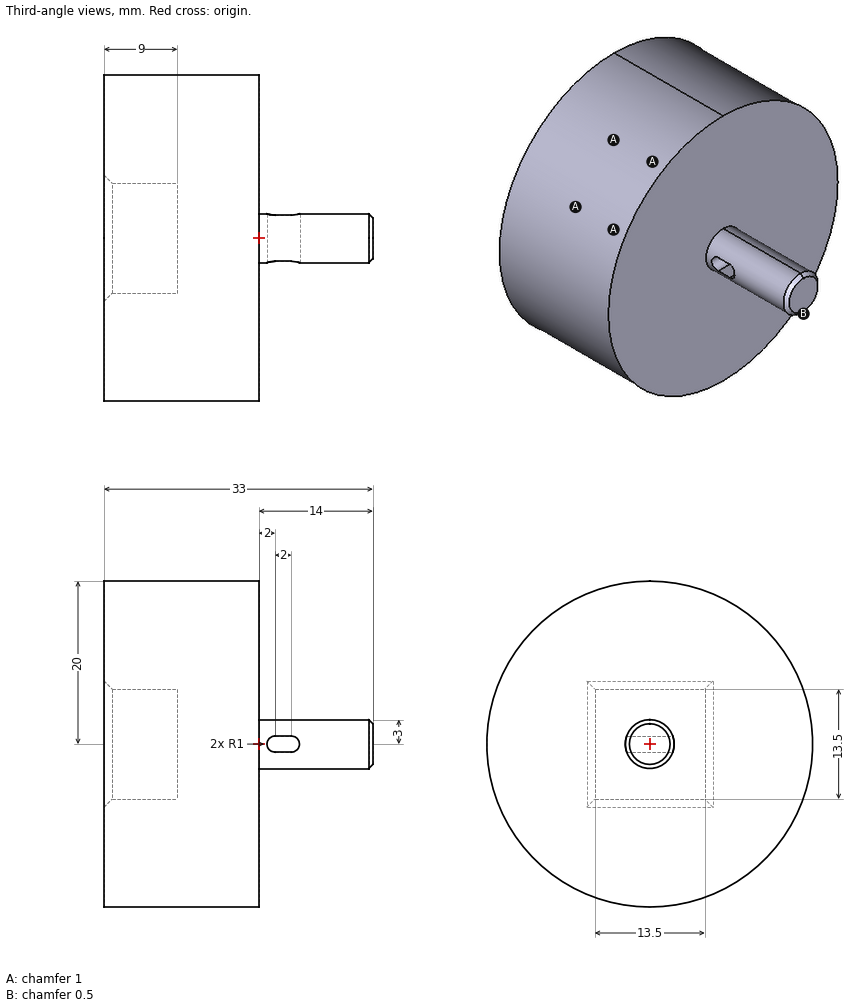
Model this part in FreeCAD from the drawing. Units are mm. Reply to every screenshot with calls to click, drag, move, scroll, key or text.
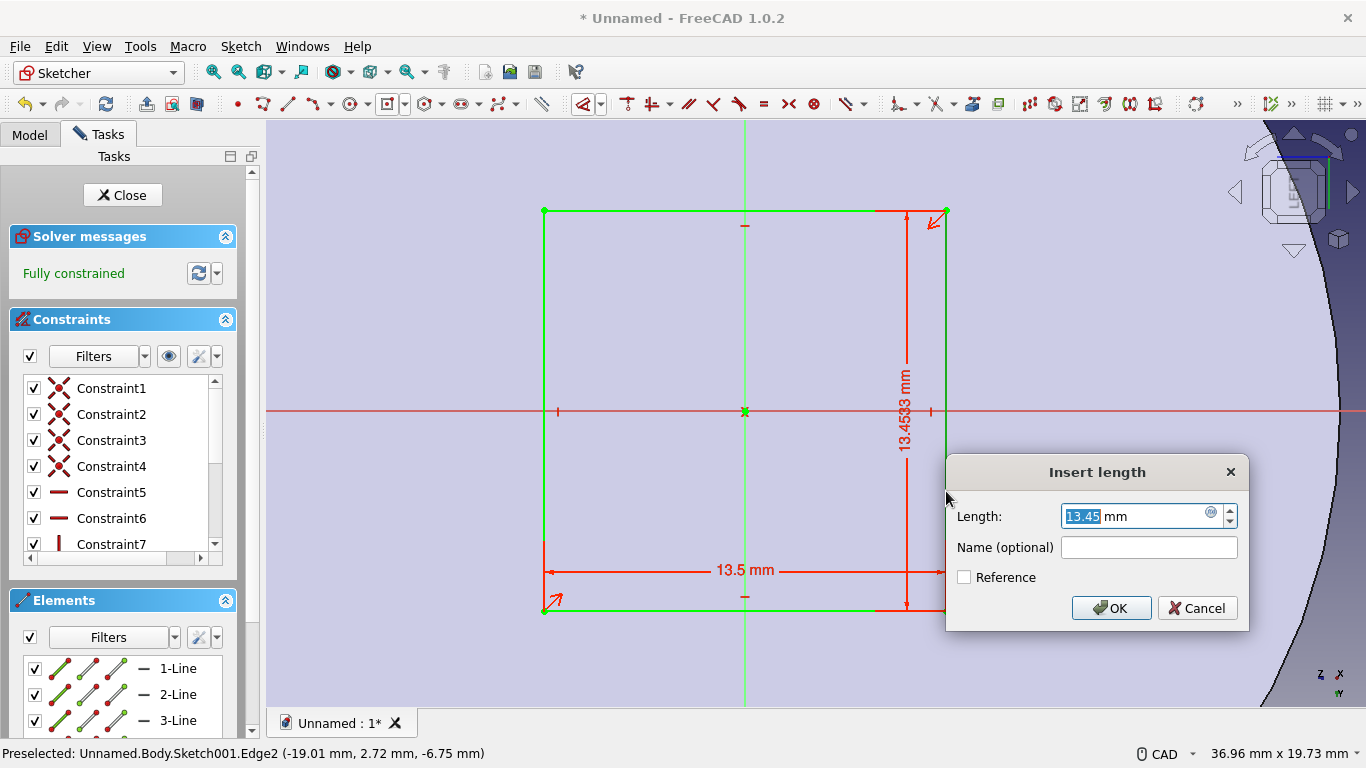
text(13.5)
key(Return)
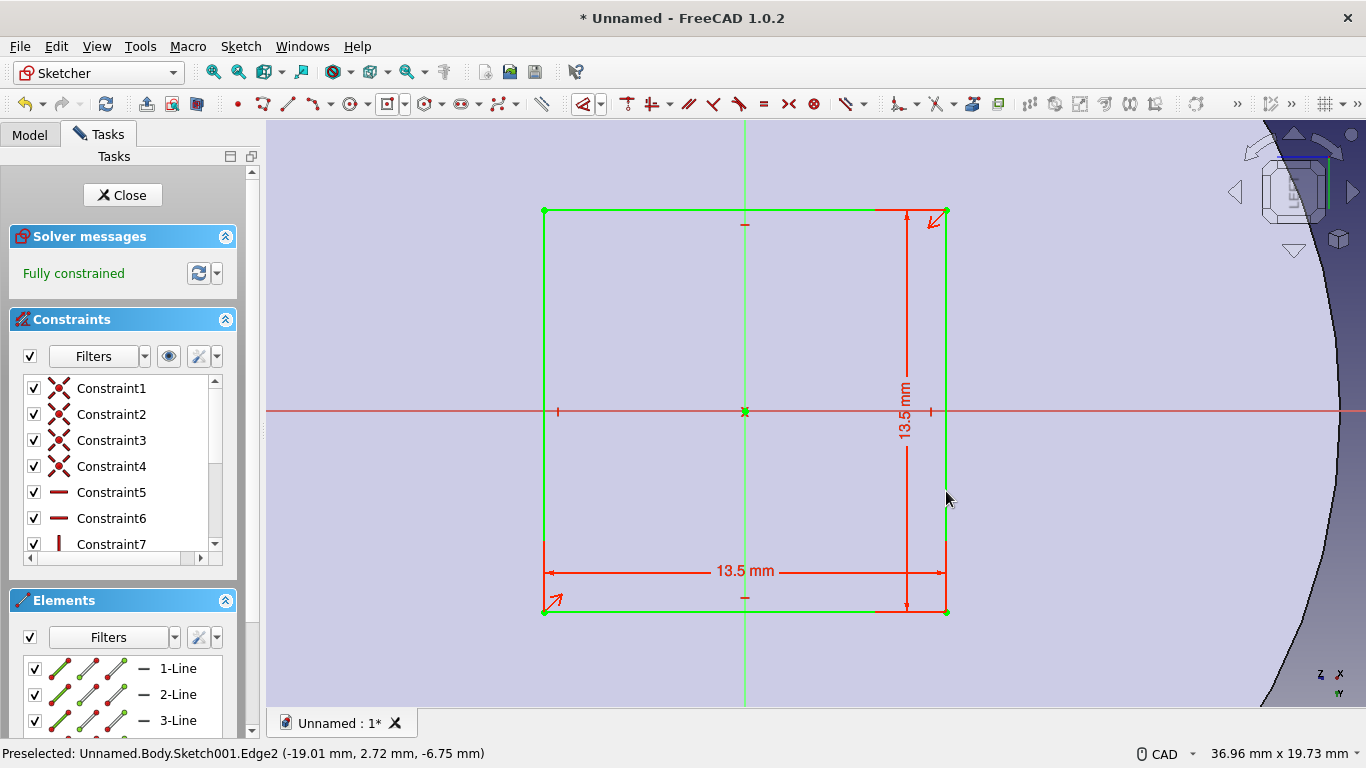
click(123, 195)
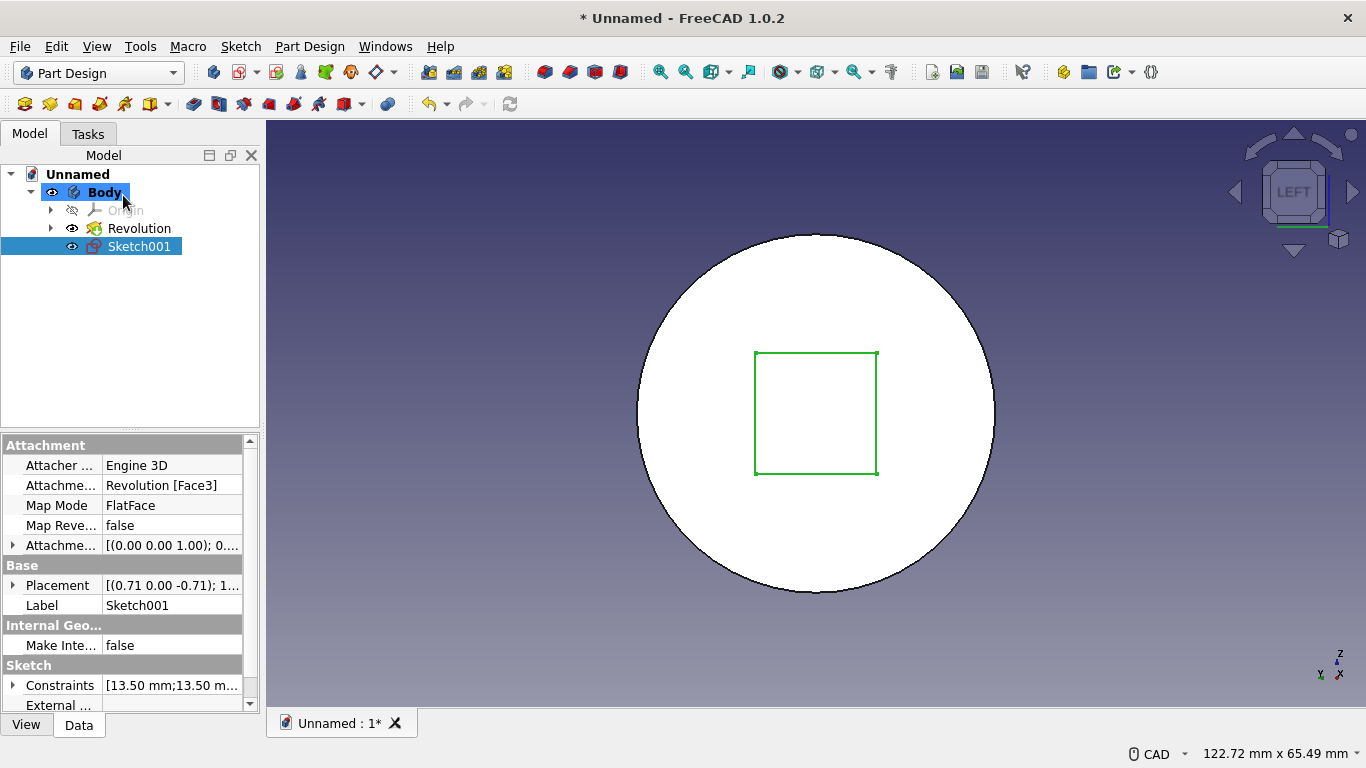
click(194, 104)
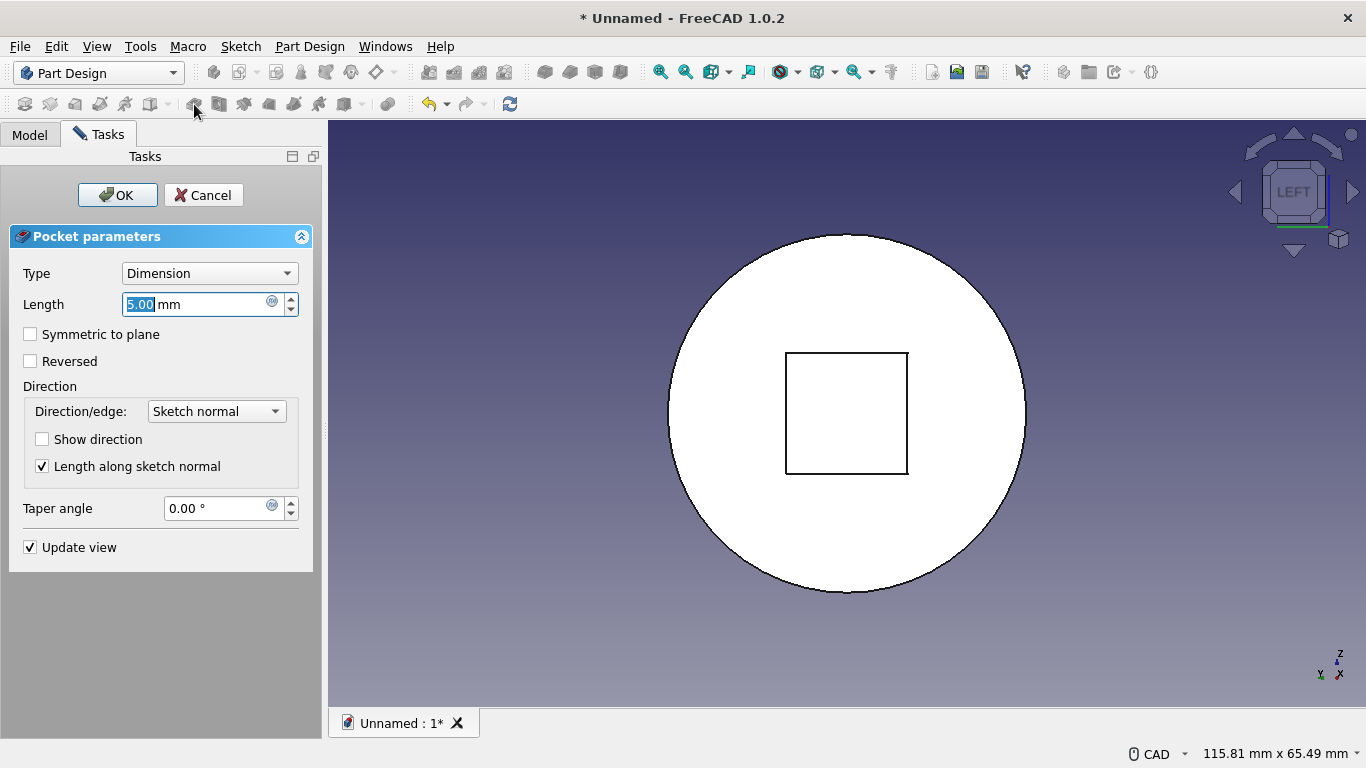
text(9)
key(Tab)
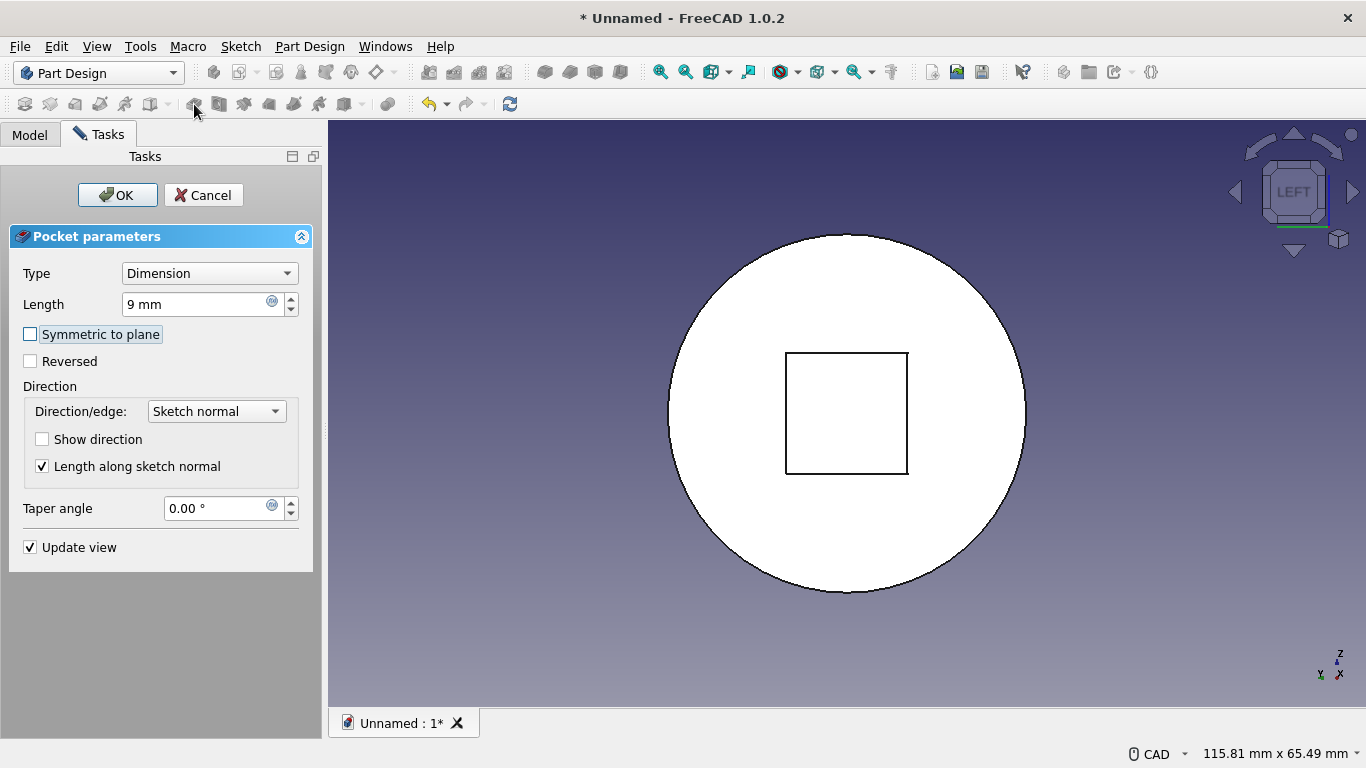
click(118, 195)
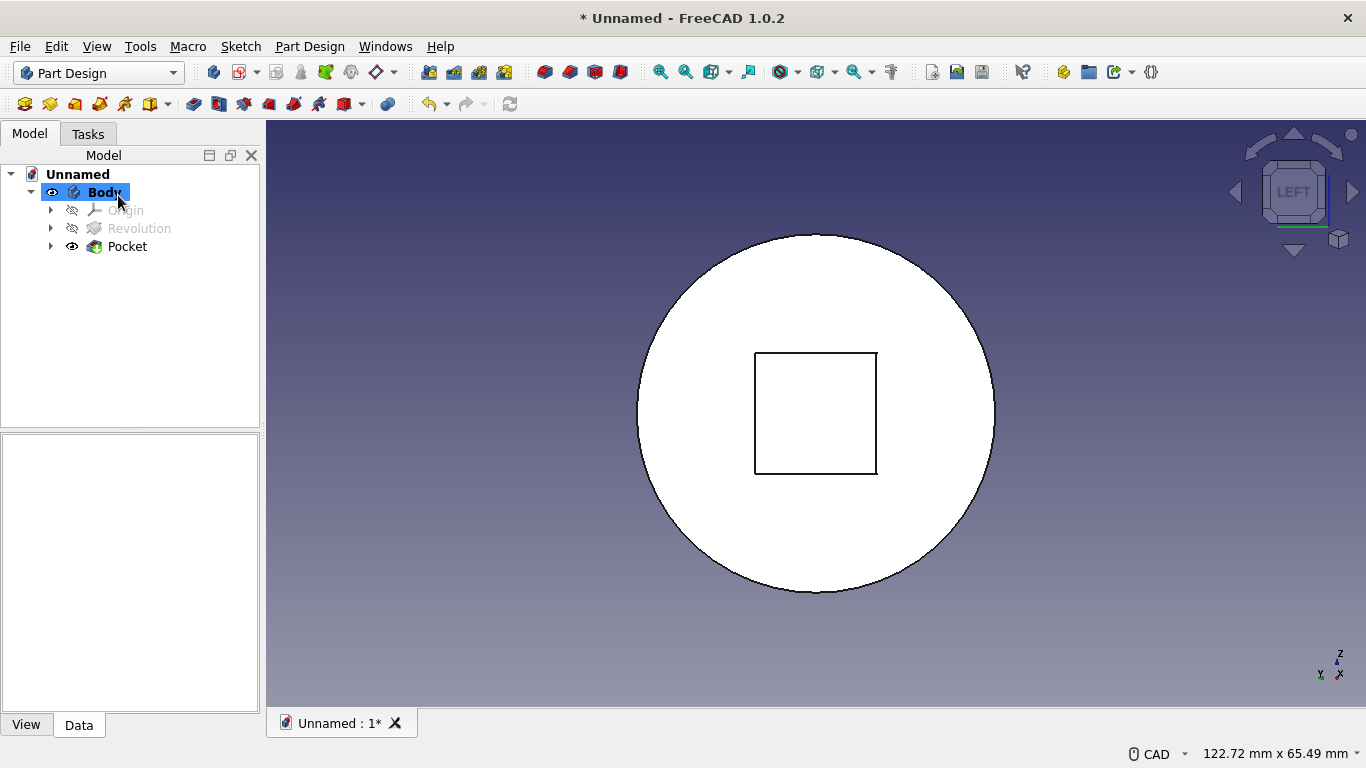
click(816, 352)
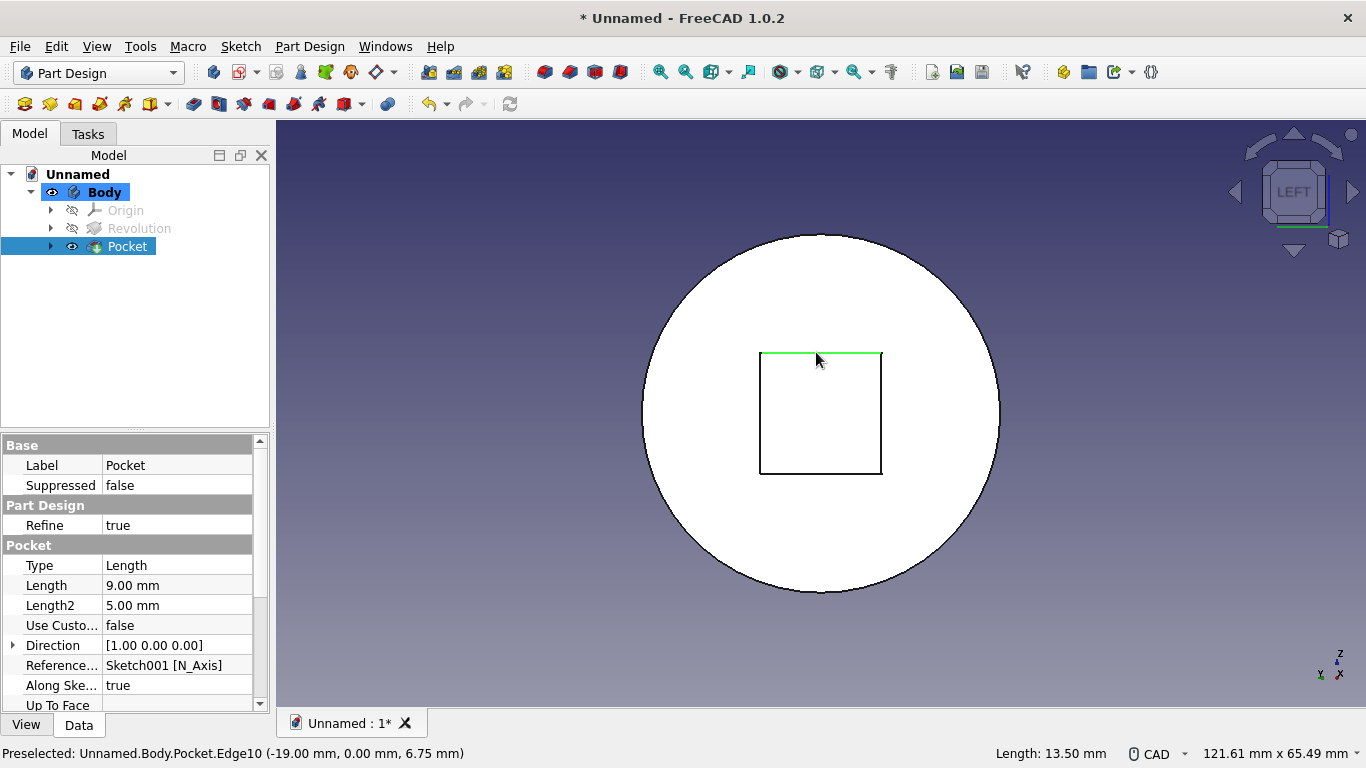
click(882, 412, ctrl)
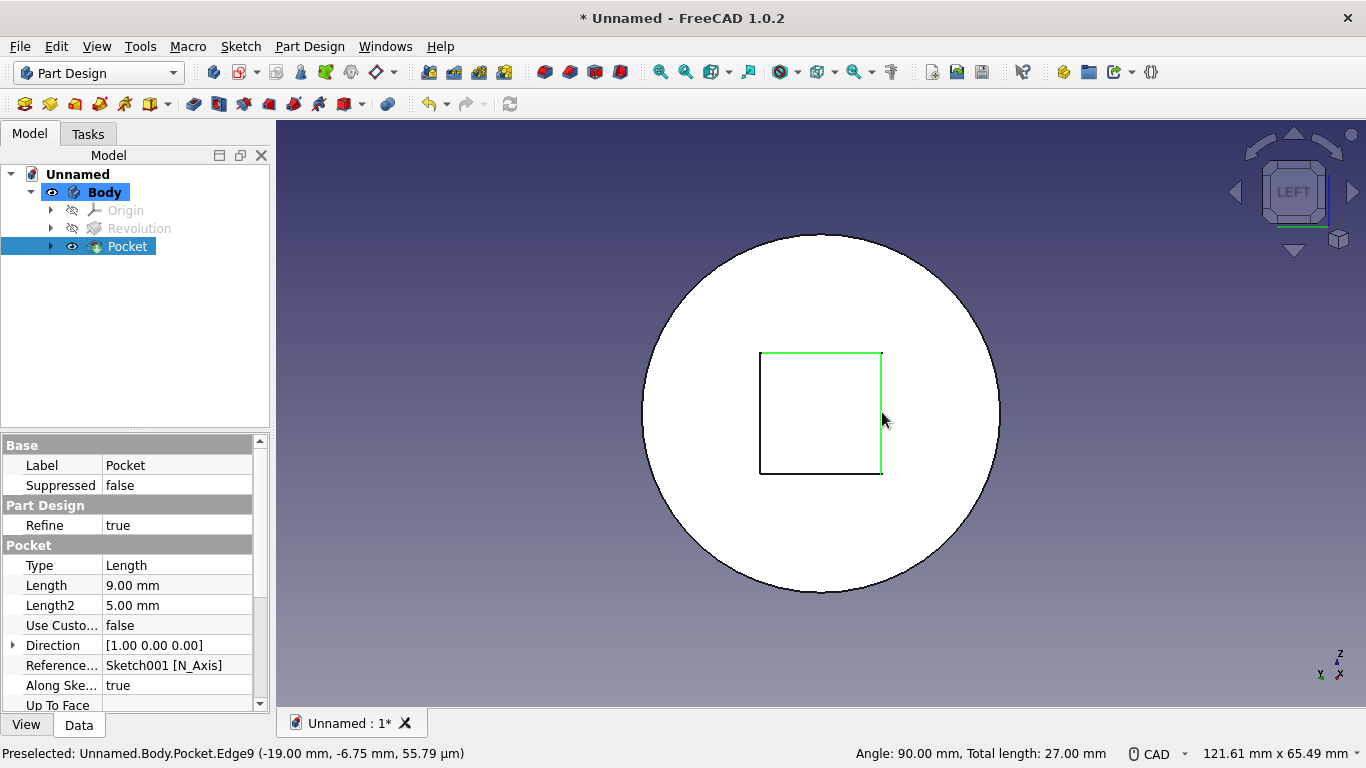
click(821, 473, ctrl)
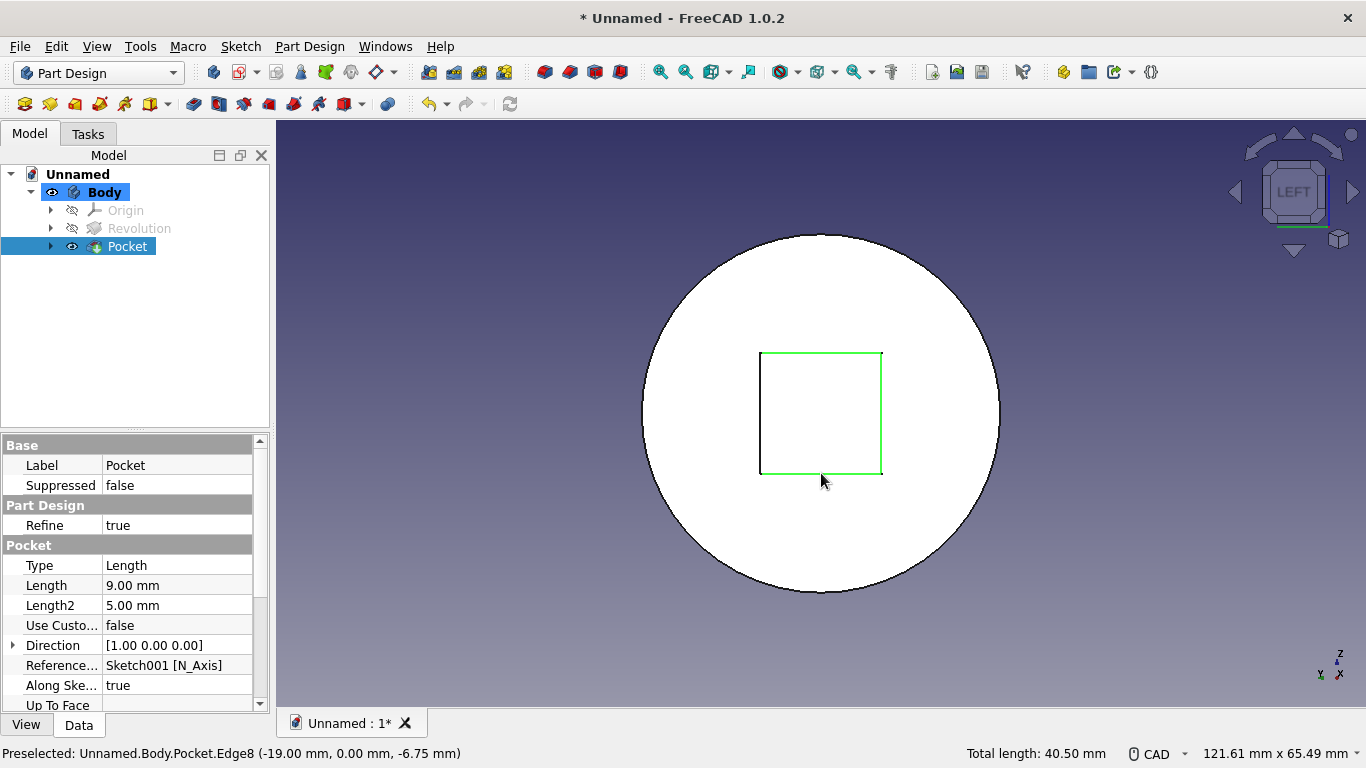
click(760, 412, ctrl)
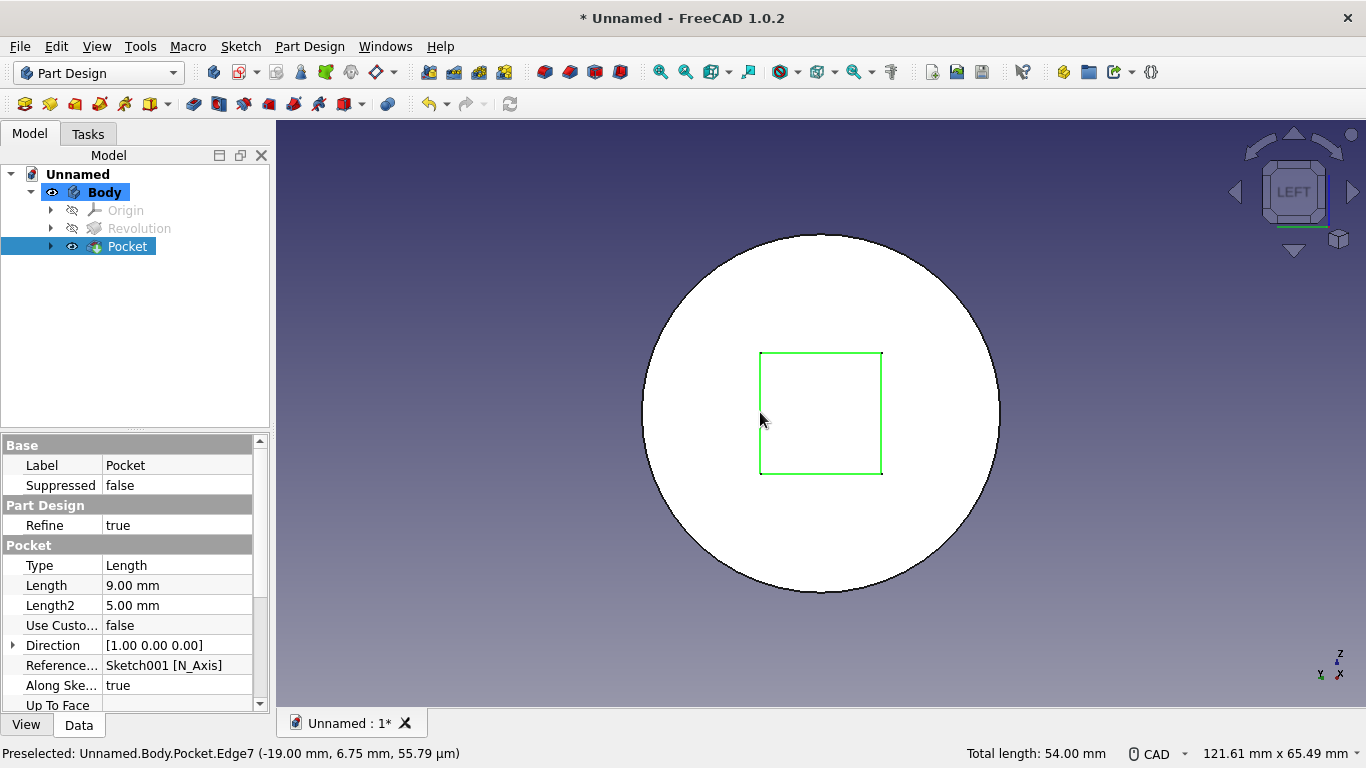
click(570, 72)